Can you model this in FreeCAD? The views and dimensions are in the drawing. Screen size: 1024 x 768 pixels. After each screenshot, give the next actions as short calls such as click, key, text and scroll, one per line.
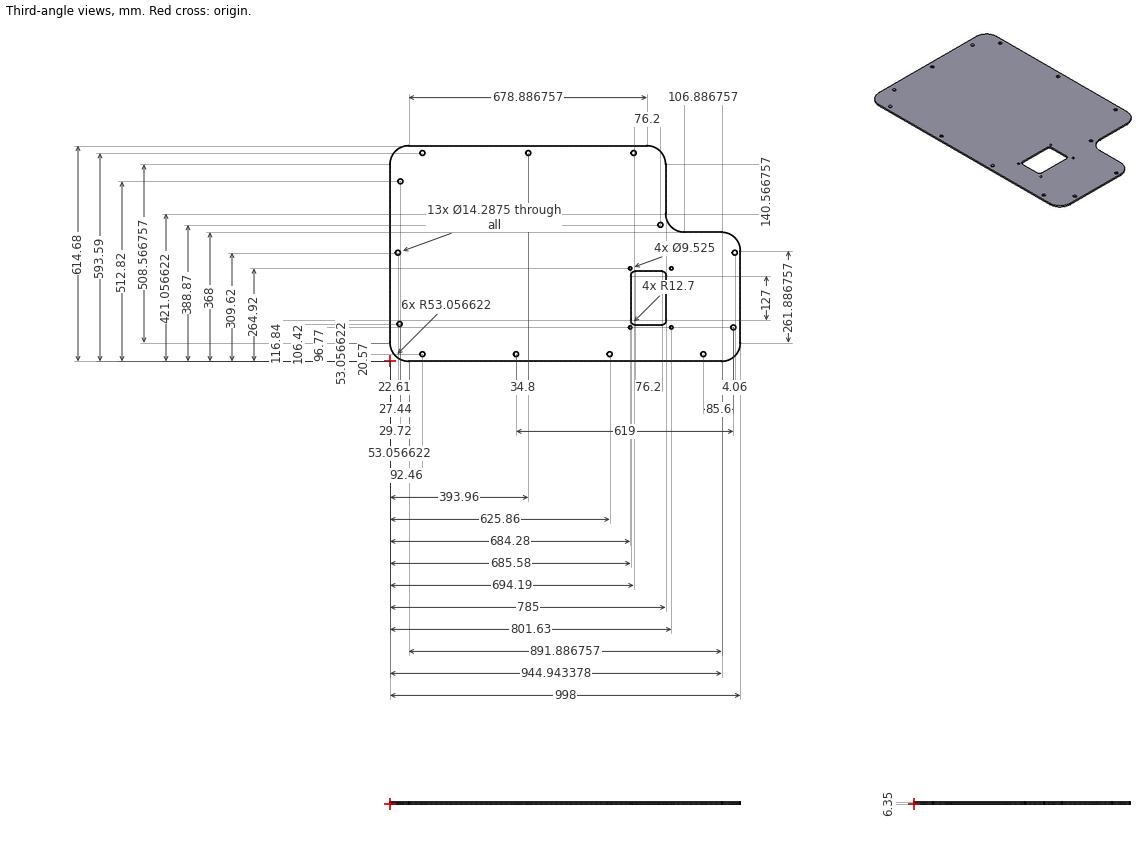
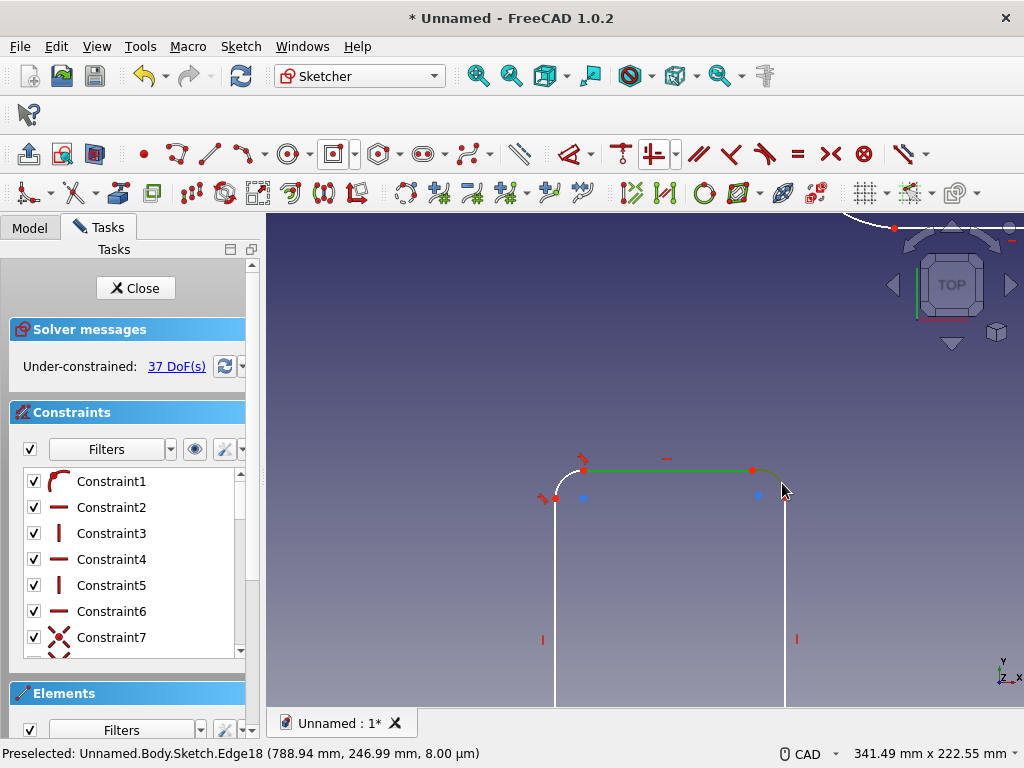
click(765, 154)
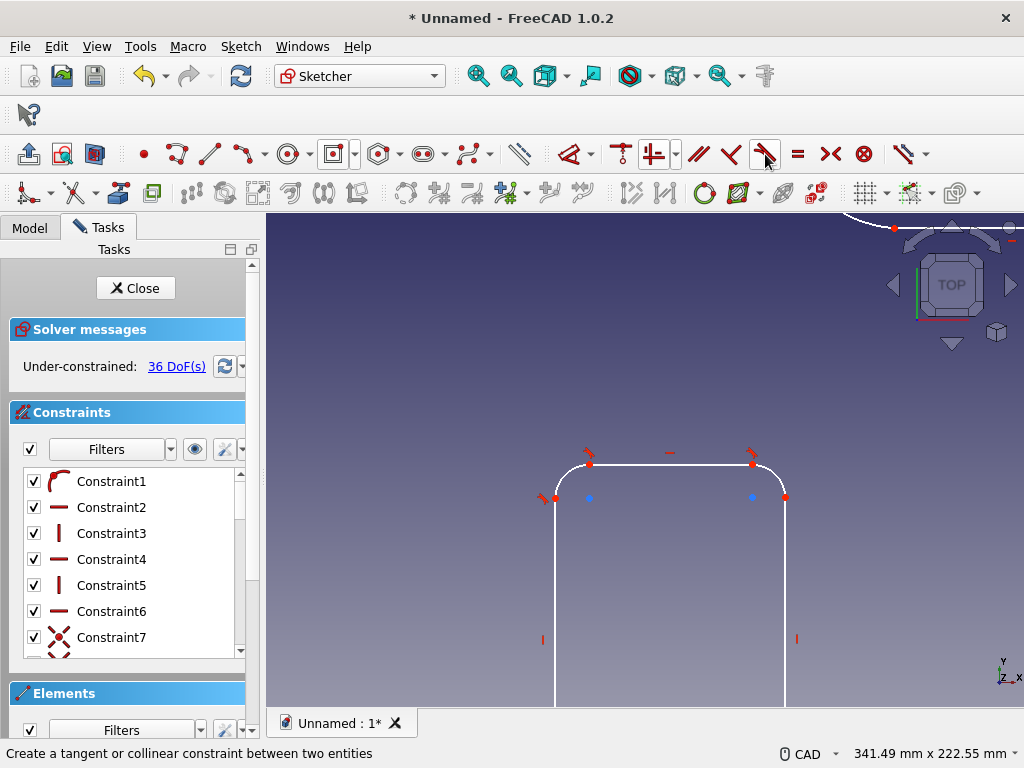
scroll(663, 481, down, 9)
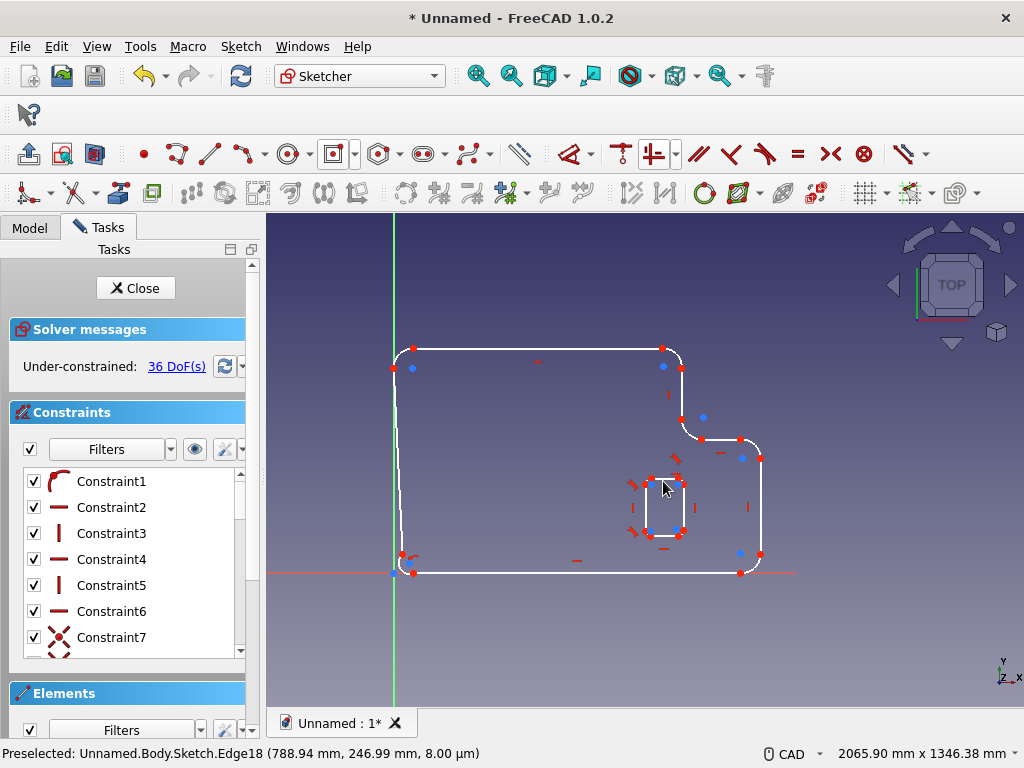
click(684, 498)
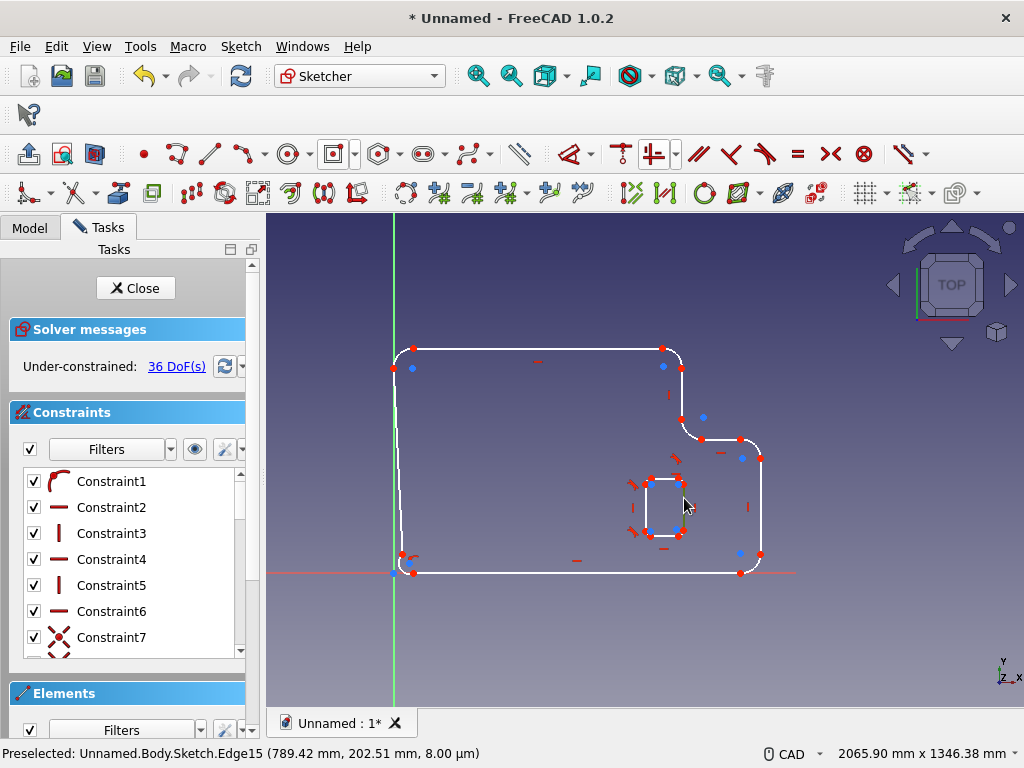
scroll(682, 480, up, 7)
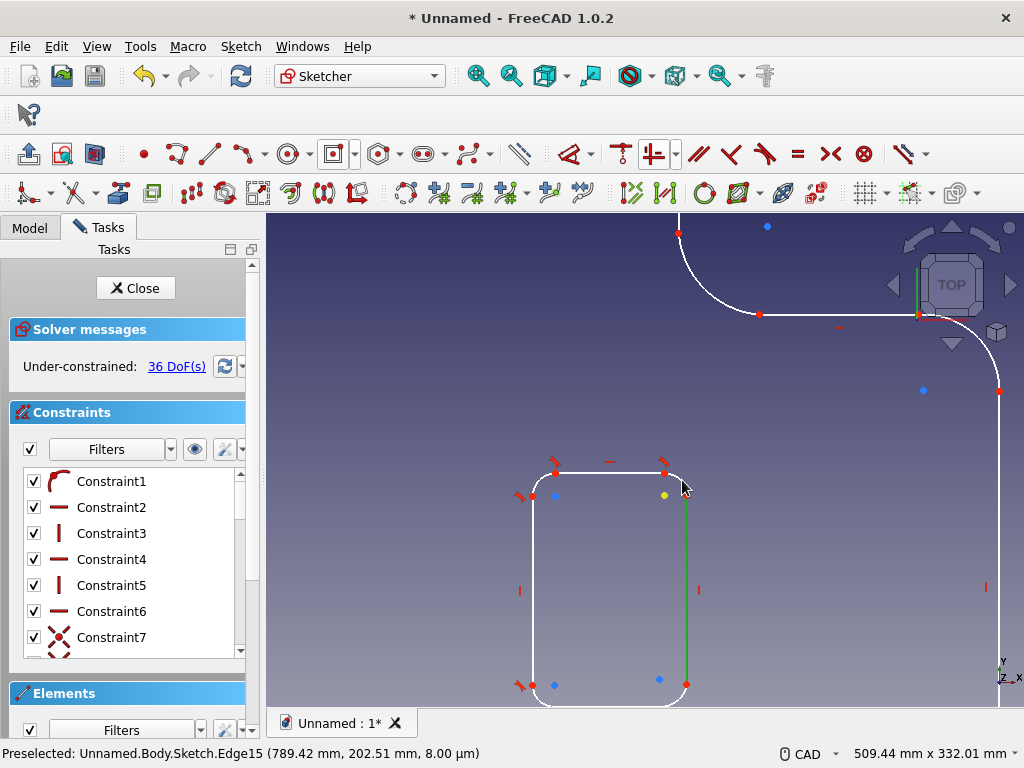
click(680, 480)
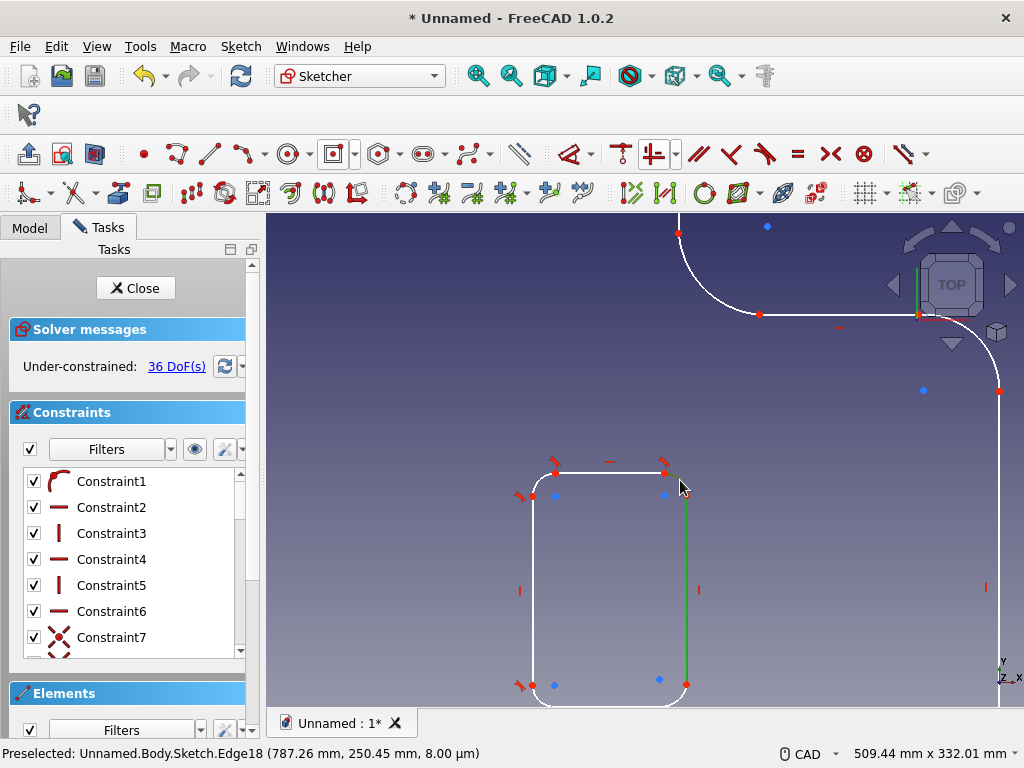
click(765, 154)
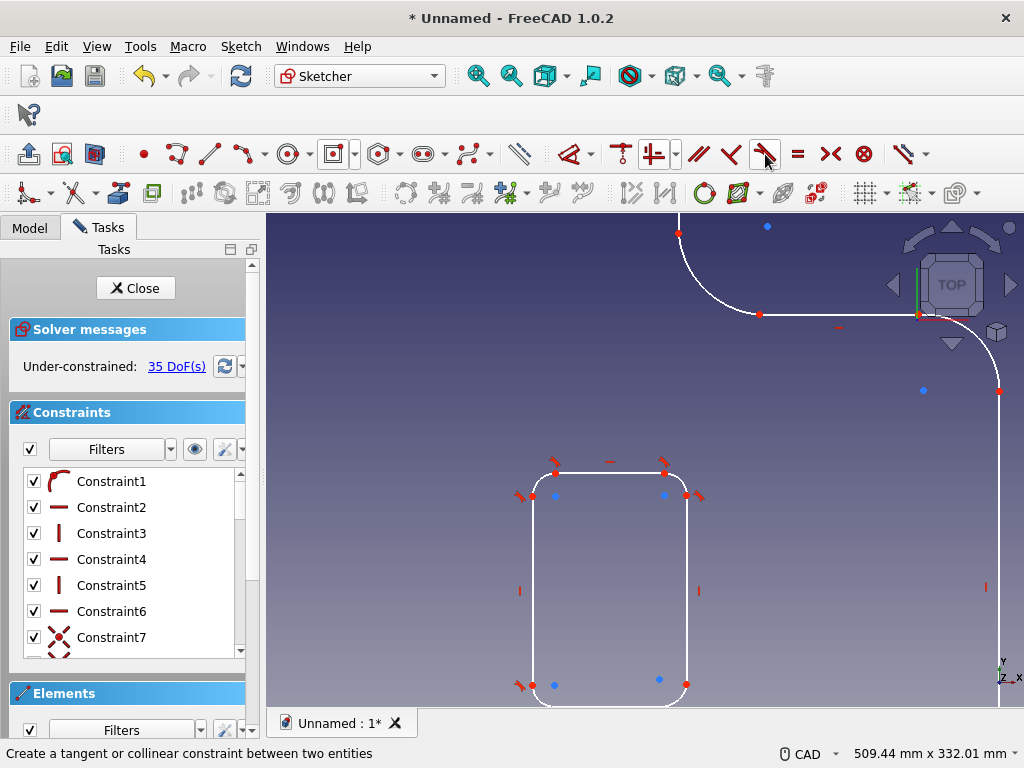
scroll(682, 480, down, 7)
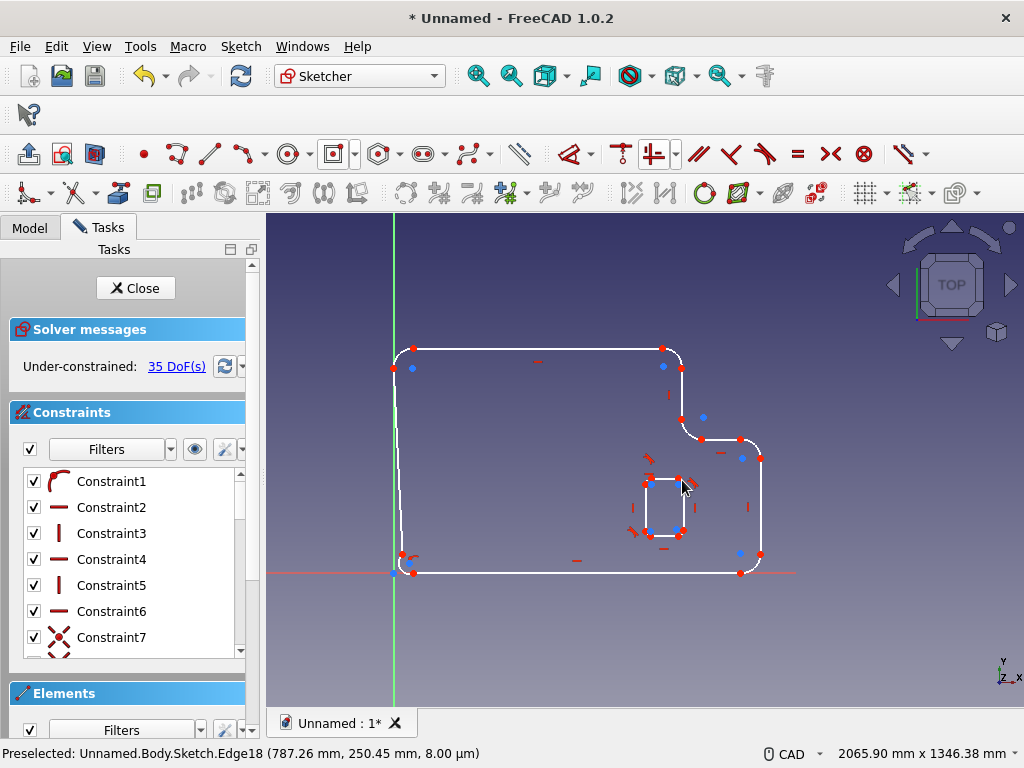
click(684, 498)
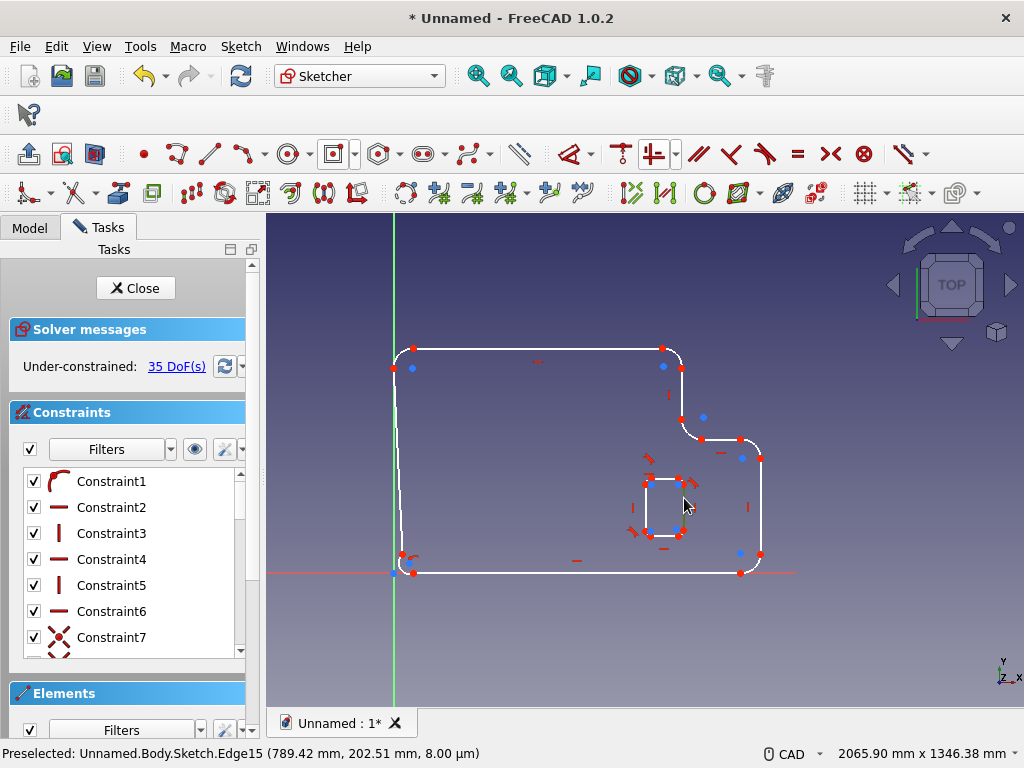
scroll(682, 534, up, 7)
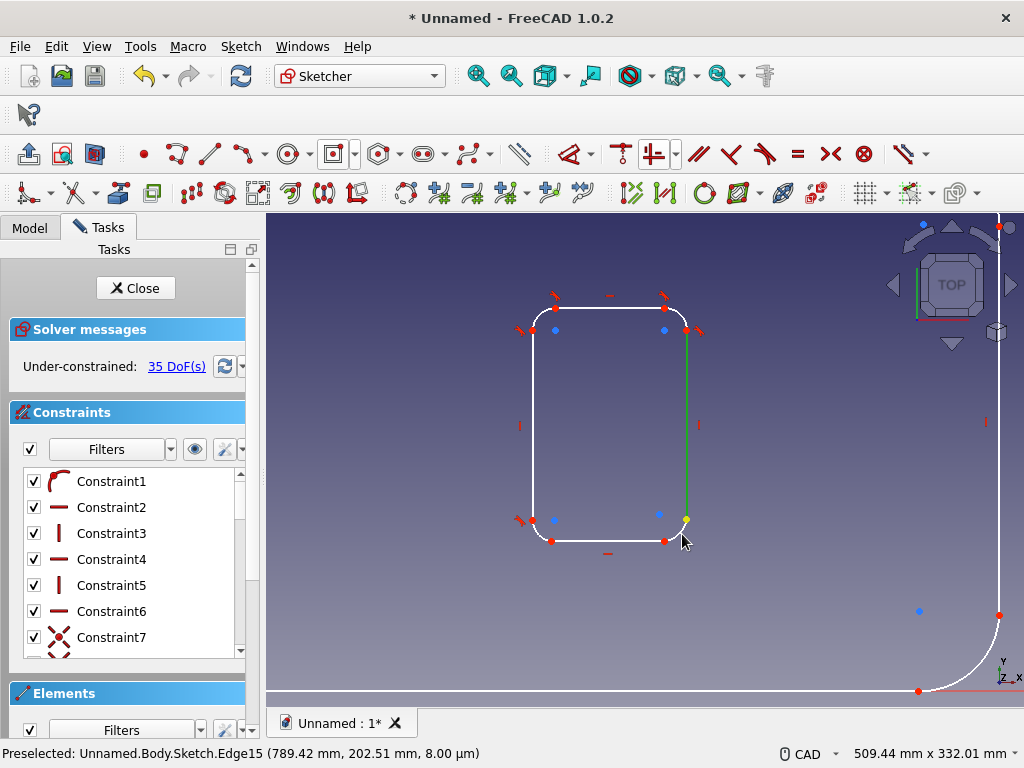
click(679, 534)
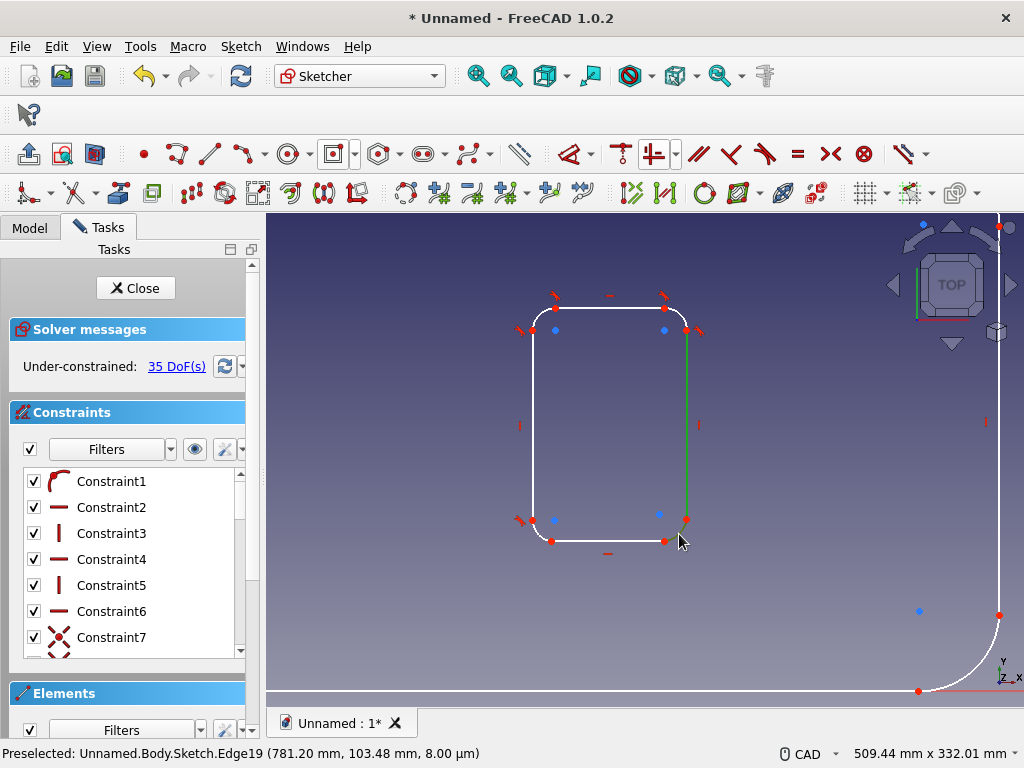
click(765, 154)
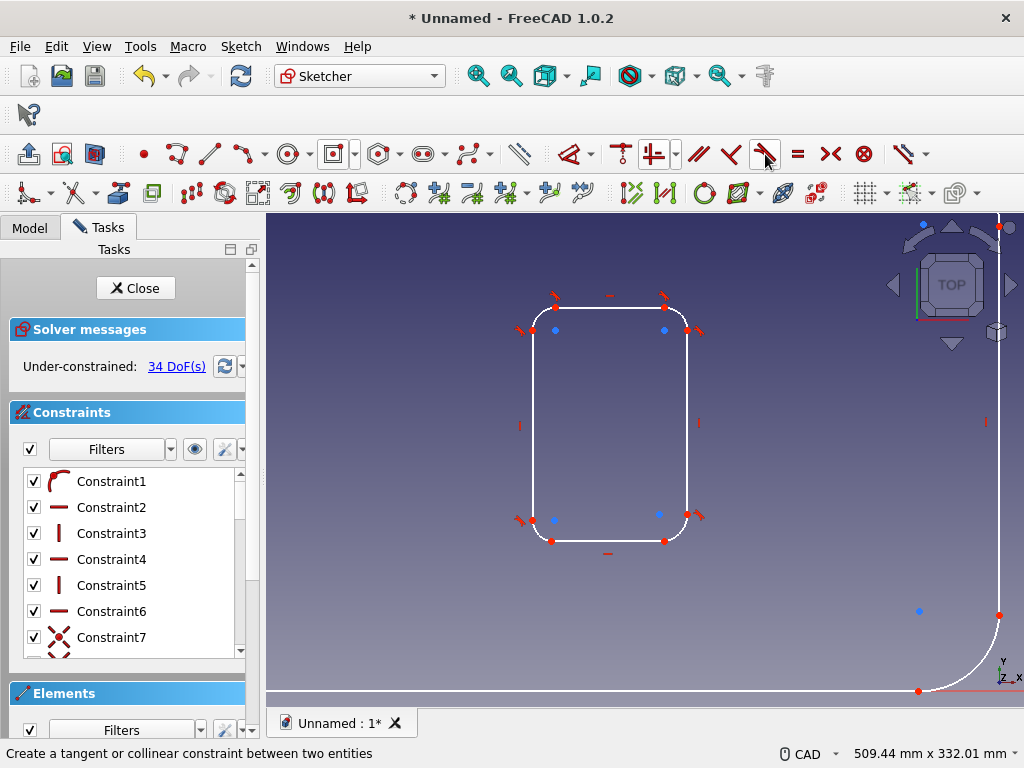
click(631, 541)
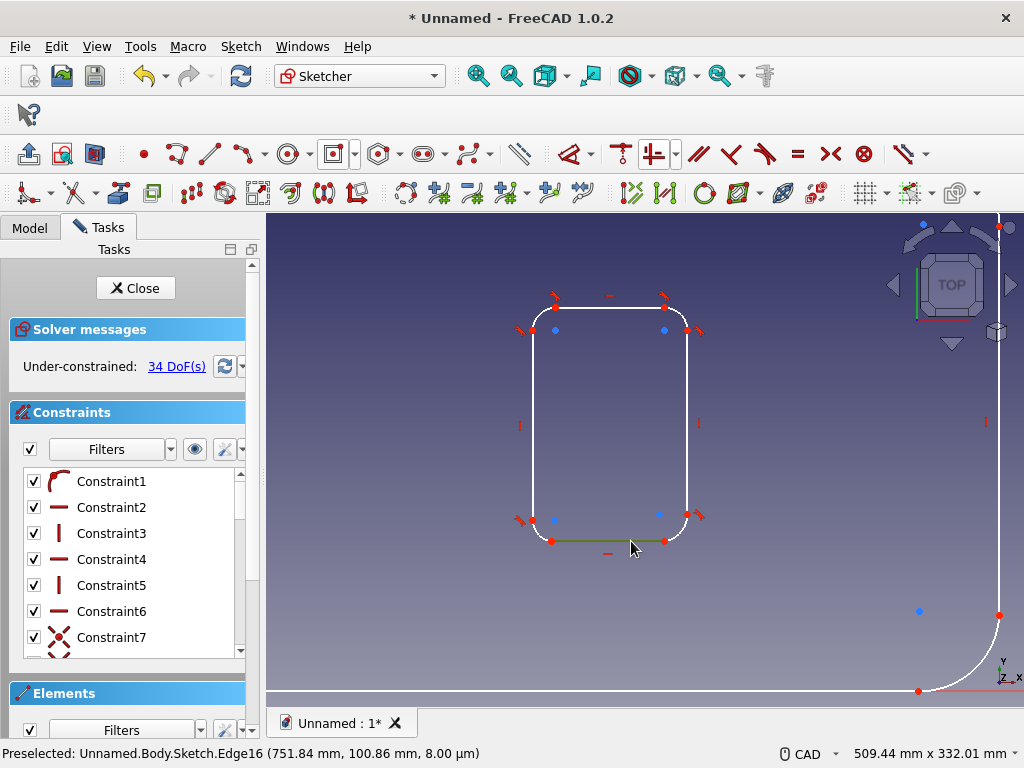
click(675, 537)